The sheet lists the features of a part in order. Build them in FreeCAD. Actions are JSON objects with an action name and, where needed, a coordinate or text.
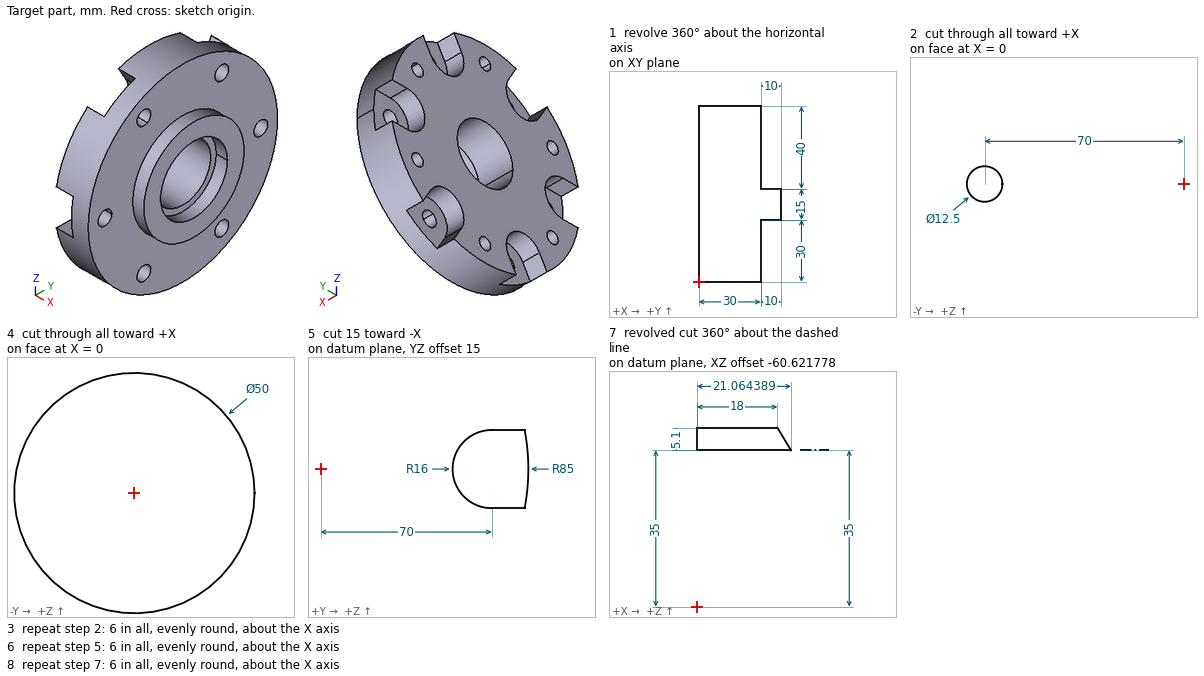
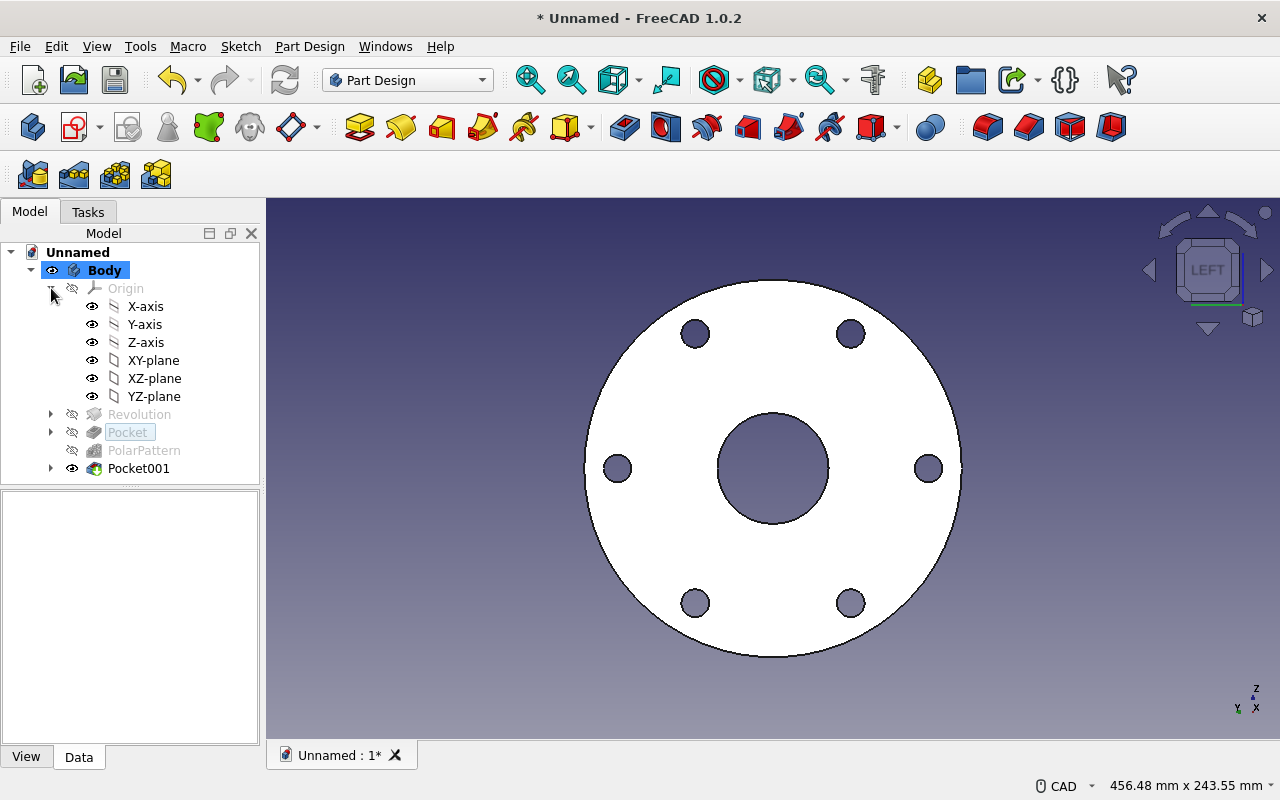
{"action": "left_click", "coordinate": [137, 396]}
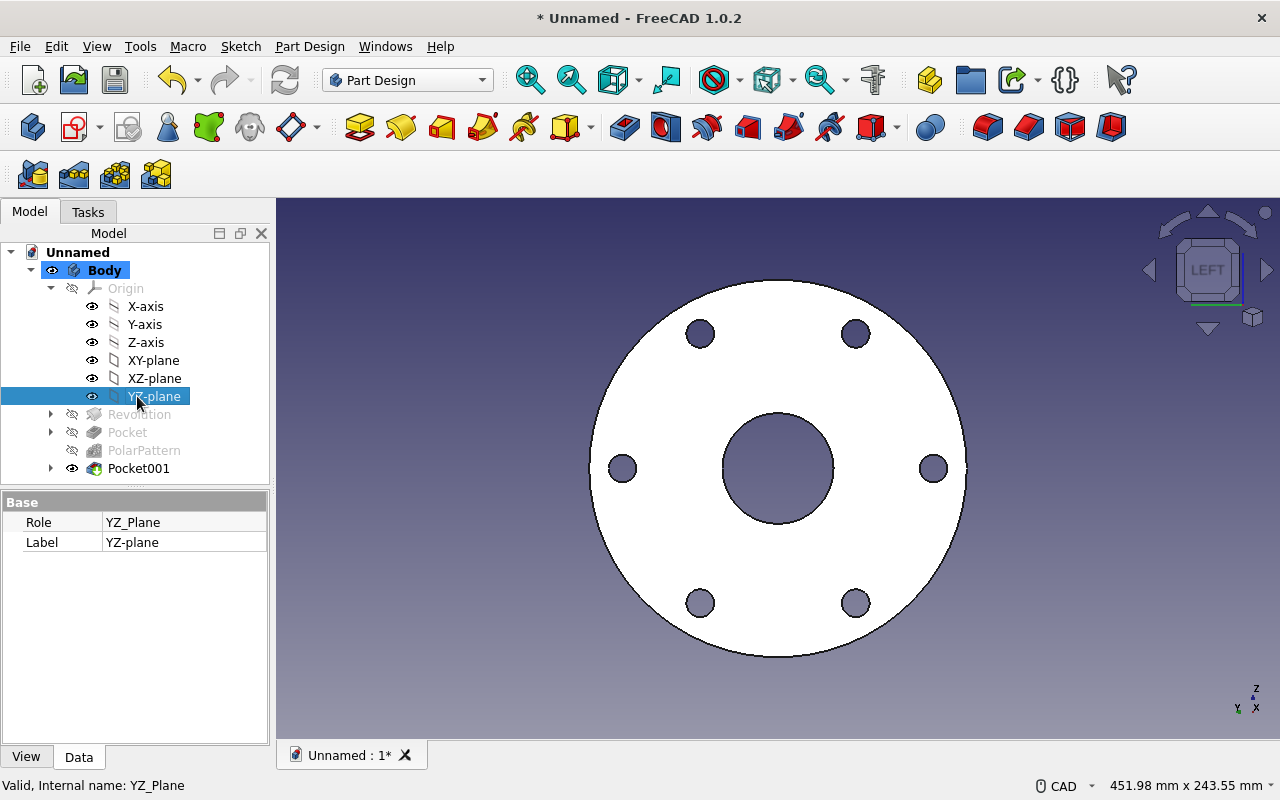
{"action": "left_click", "coordinate": [290, 128]}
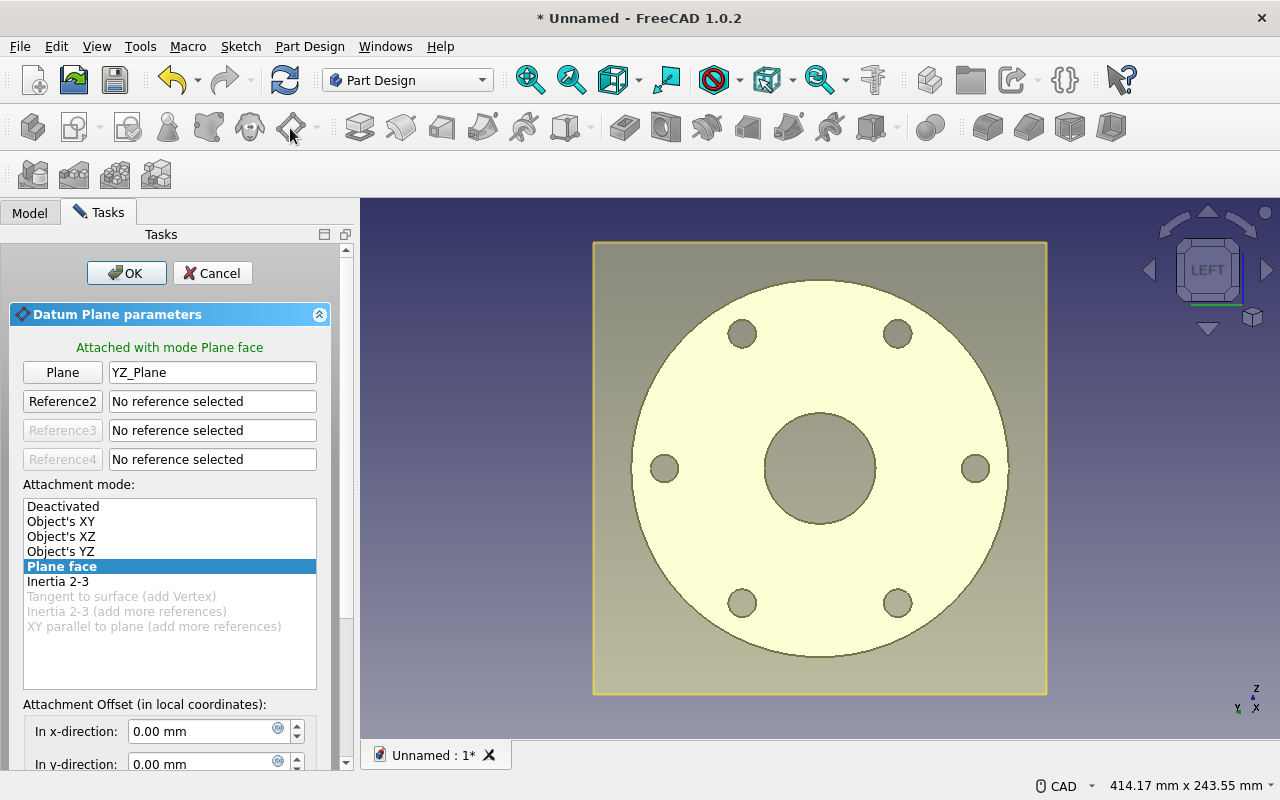
{"action": "scroll", "coordinate": [346, 507], "scroll_direction": "down", "scroll_amount": 2}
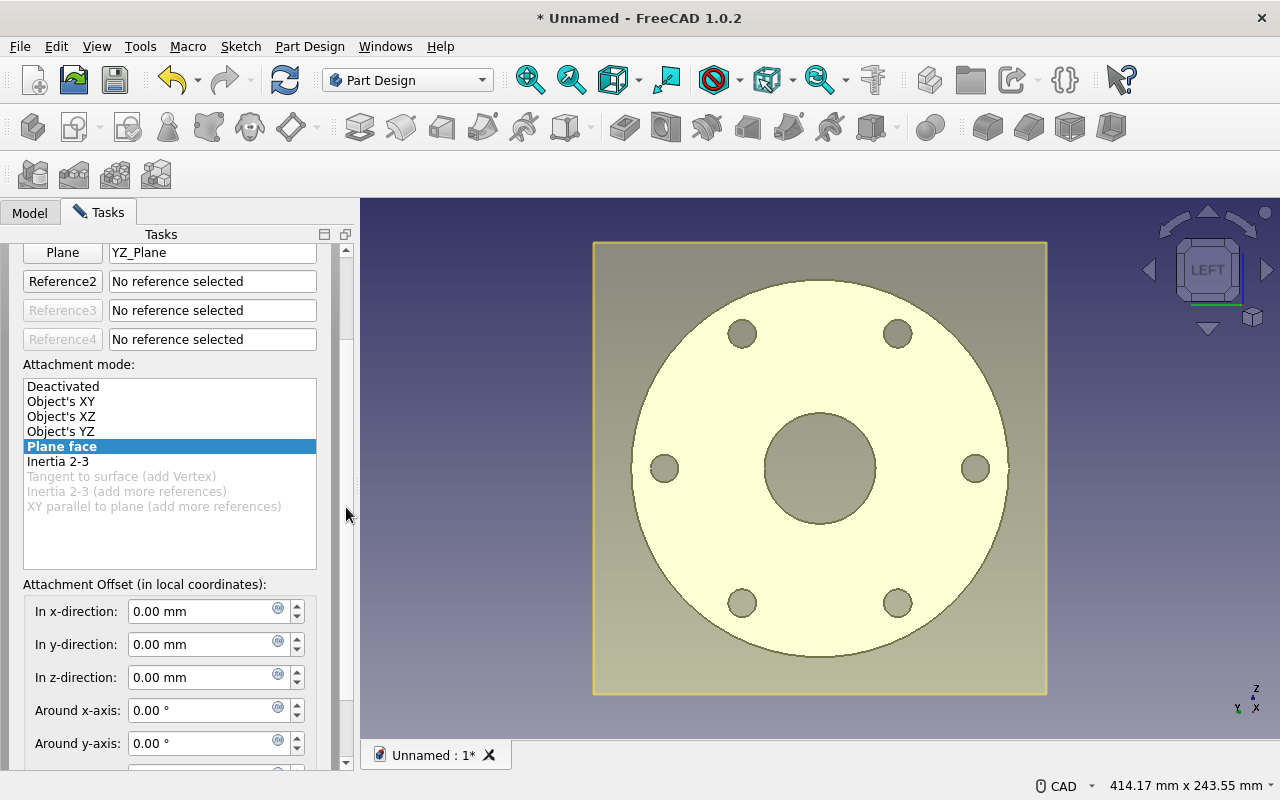
{"action": "triple_click", "coordinate": [210, 678]}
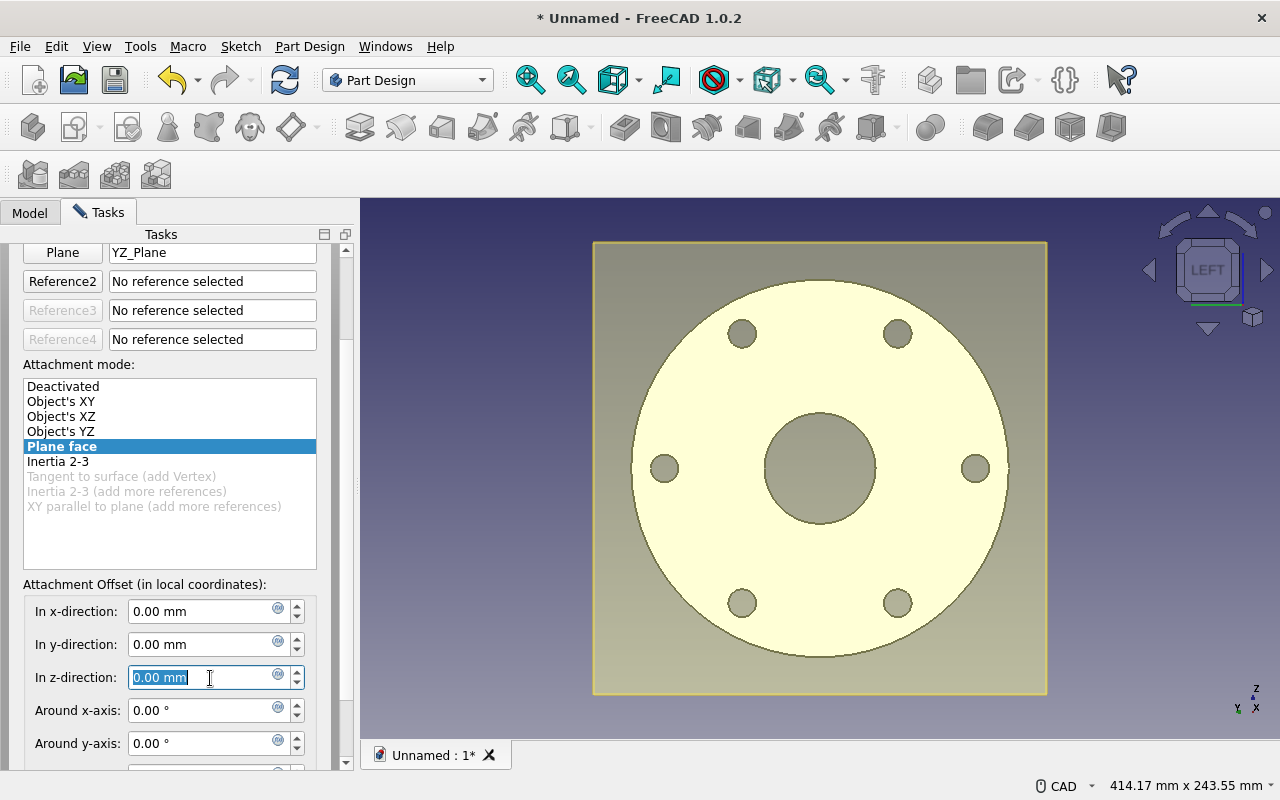
{"action": "type", "text": "15"}
{"action": "key", "text": "Tab"}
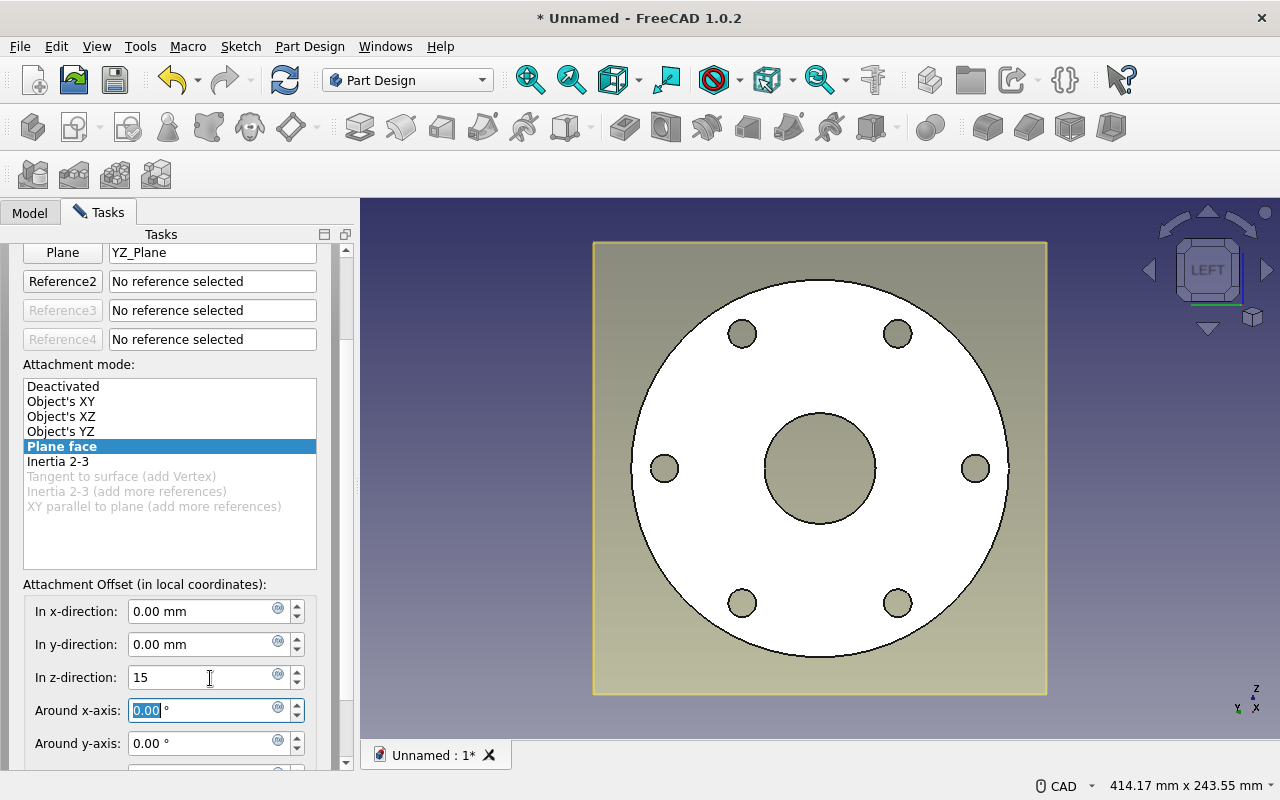
{"action": "scroll", "coordinate": [346, 507], "scroll_direction": "up", "scroll_amount": 3}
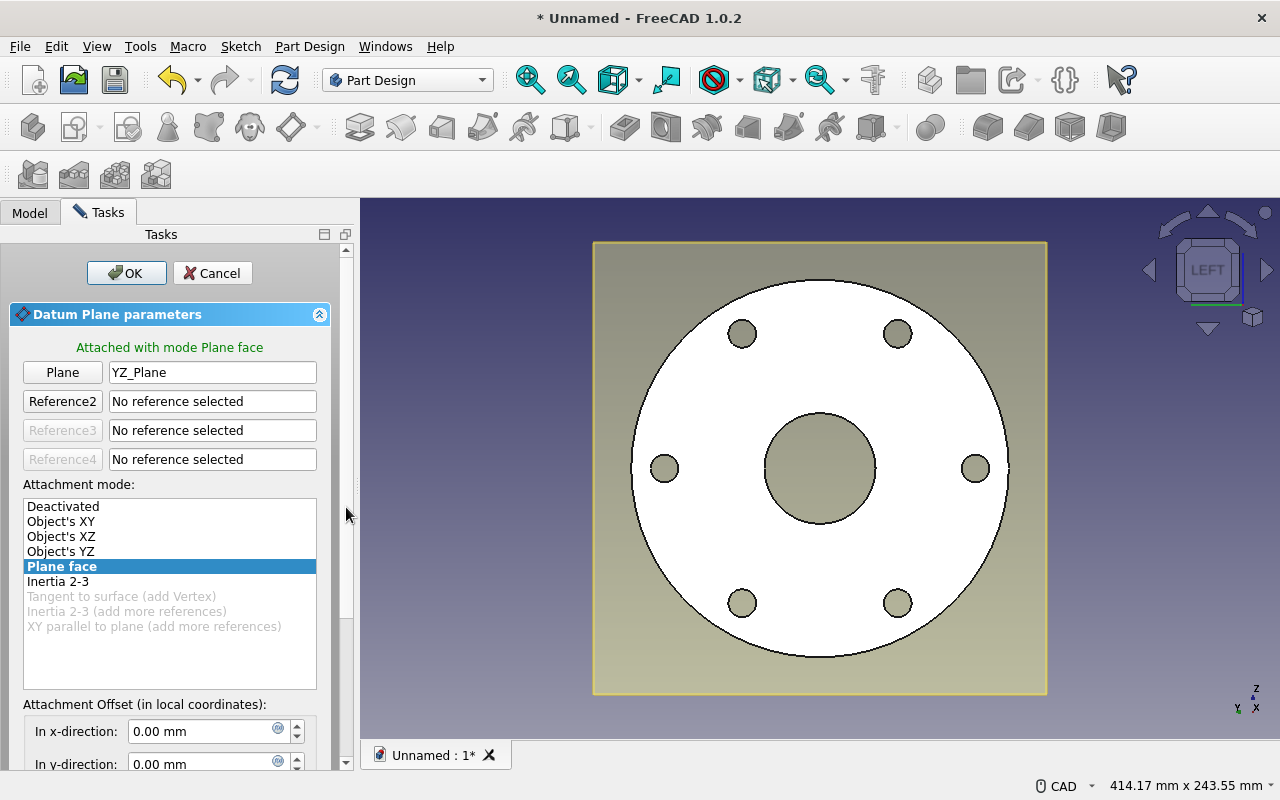
{"action": "left_click", "coordinate": [127, 273]}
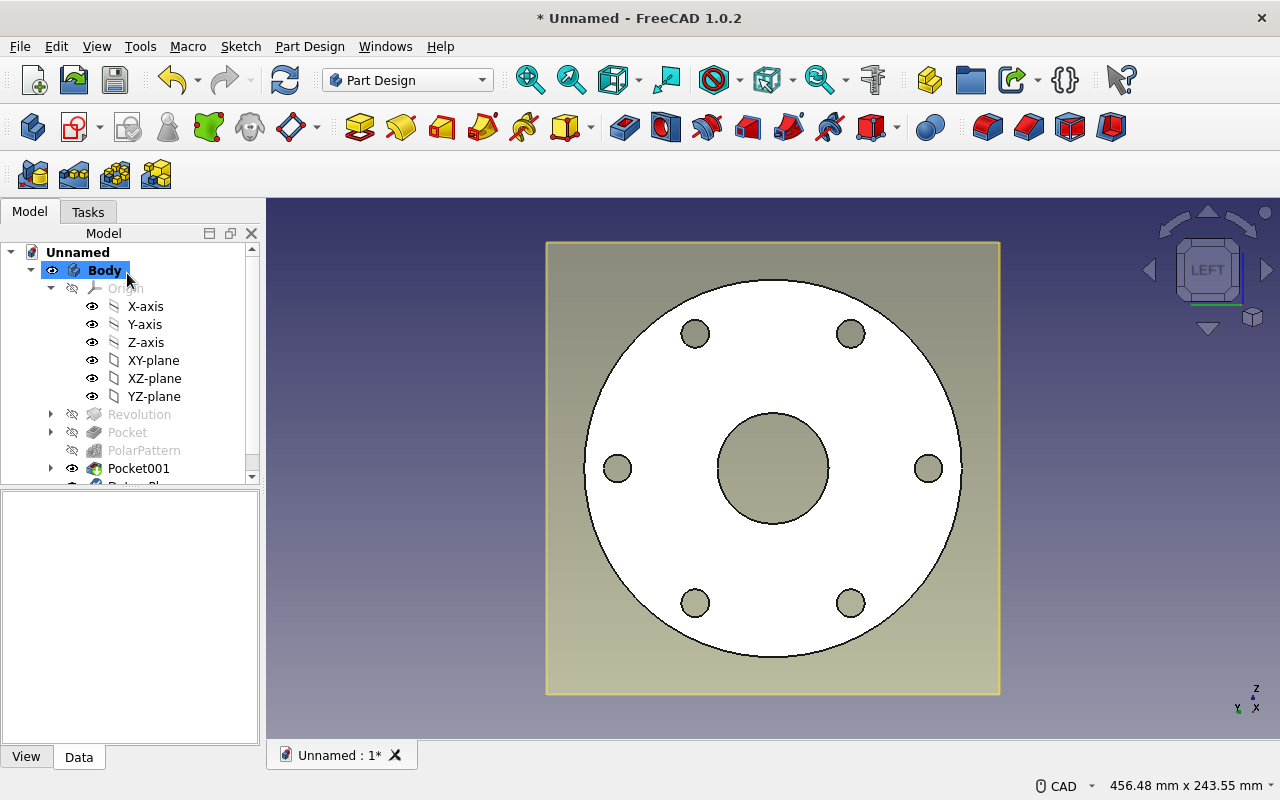
{"action": "scroll", "coordinate": [101, 356], "scroll_direction": "down", "scroll_amount": 3}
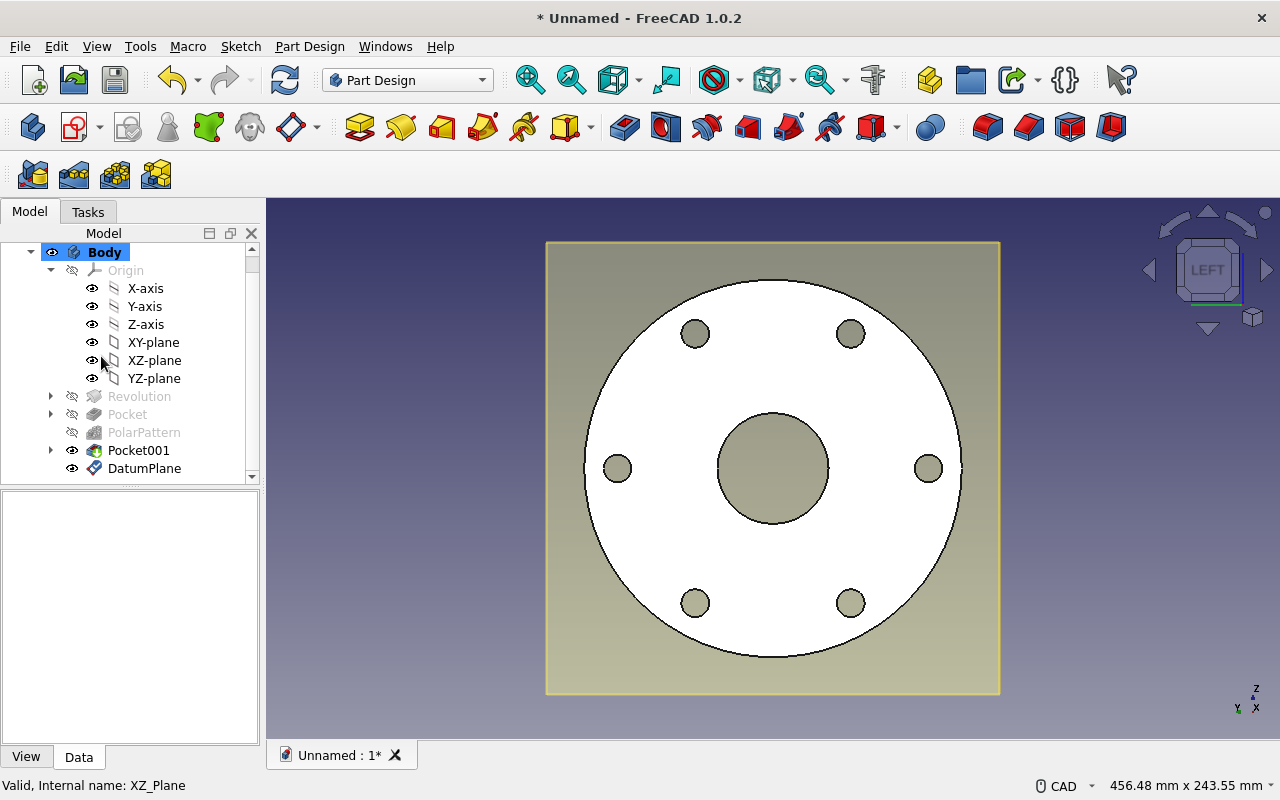
{"action": "left_click", "coordinate": [117, 468]}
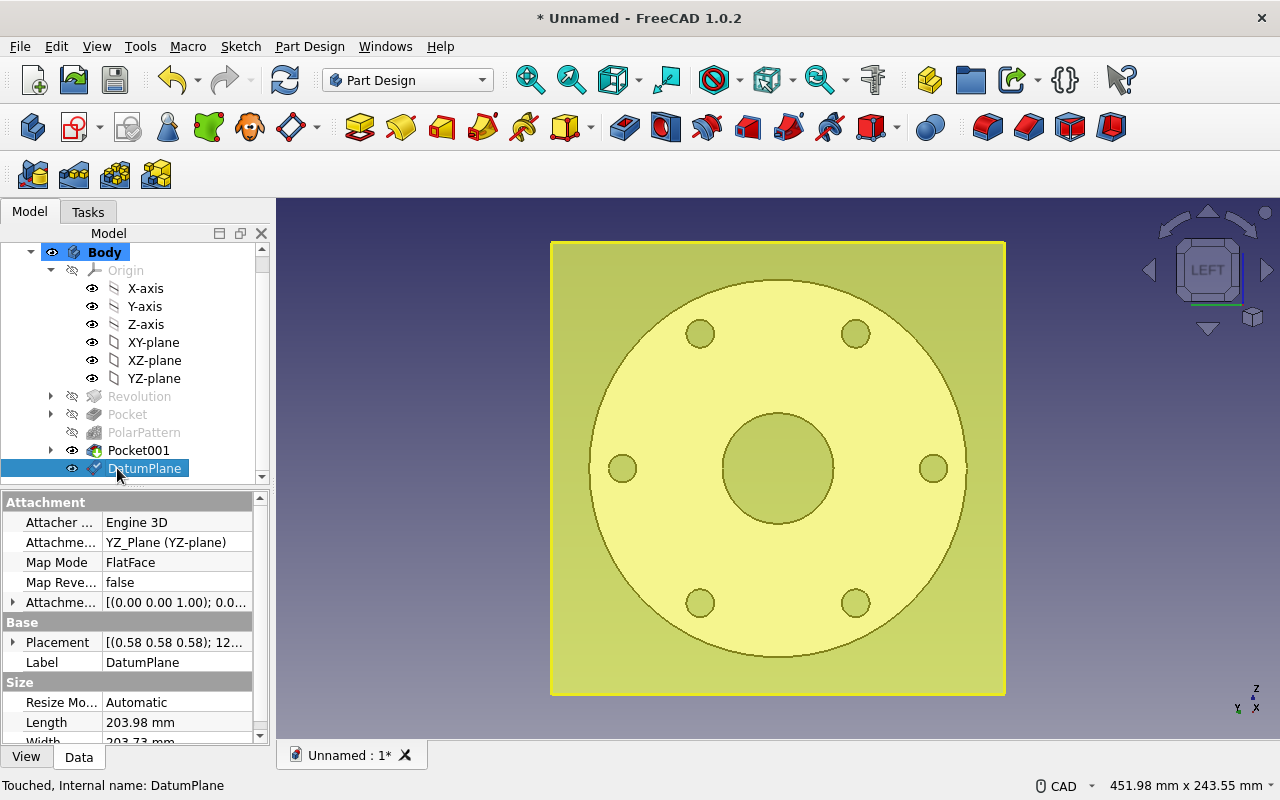
{"action": "left_click", "coordinate": [74, 128]}